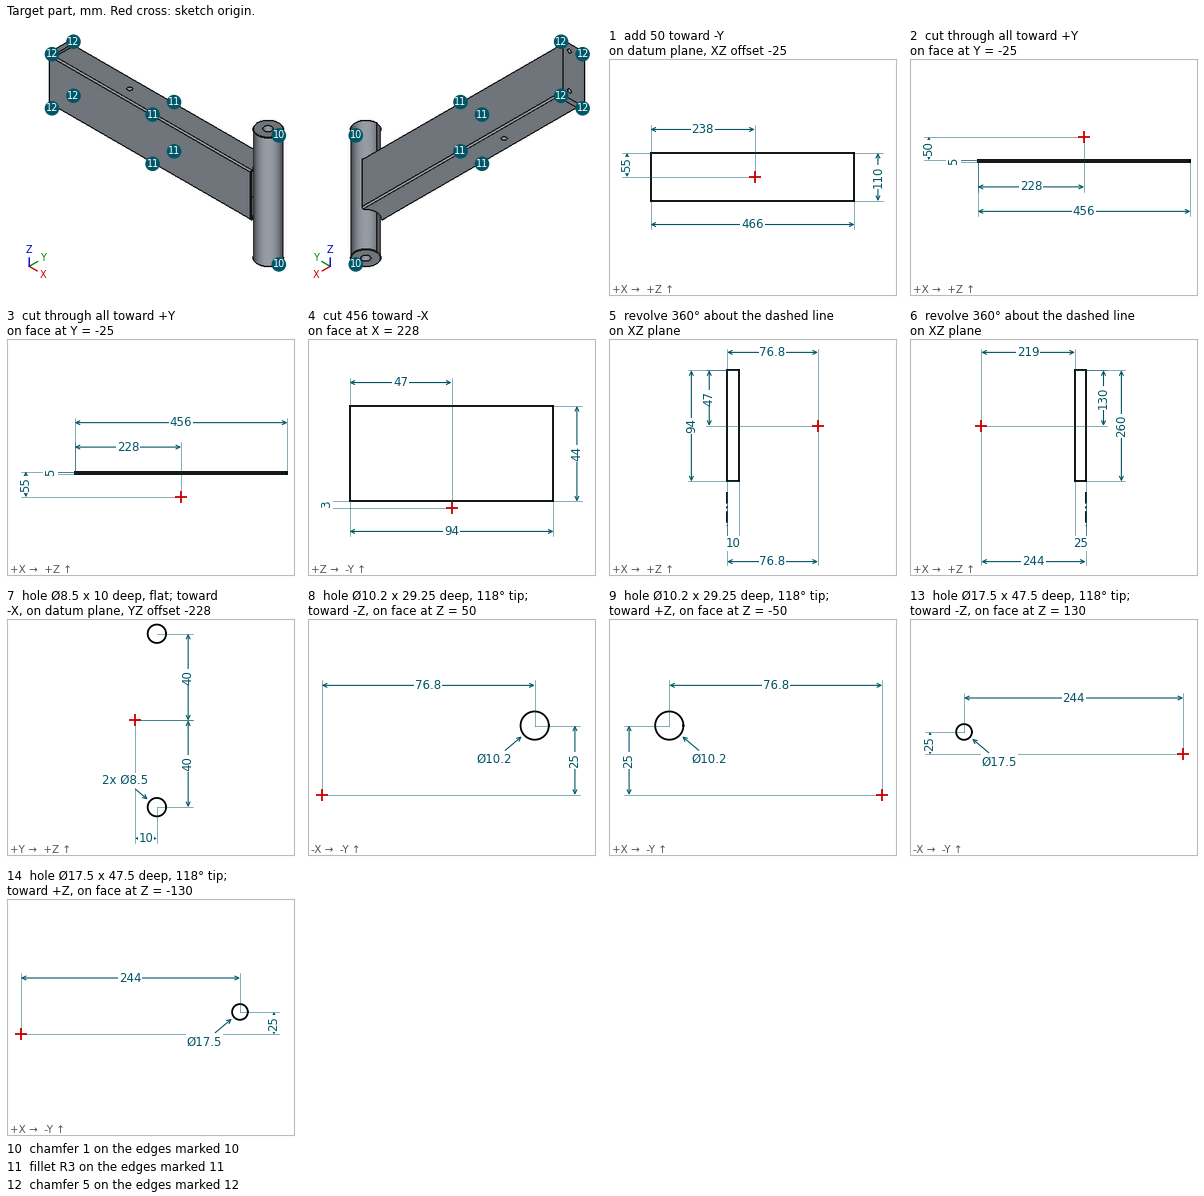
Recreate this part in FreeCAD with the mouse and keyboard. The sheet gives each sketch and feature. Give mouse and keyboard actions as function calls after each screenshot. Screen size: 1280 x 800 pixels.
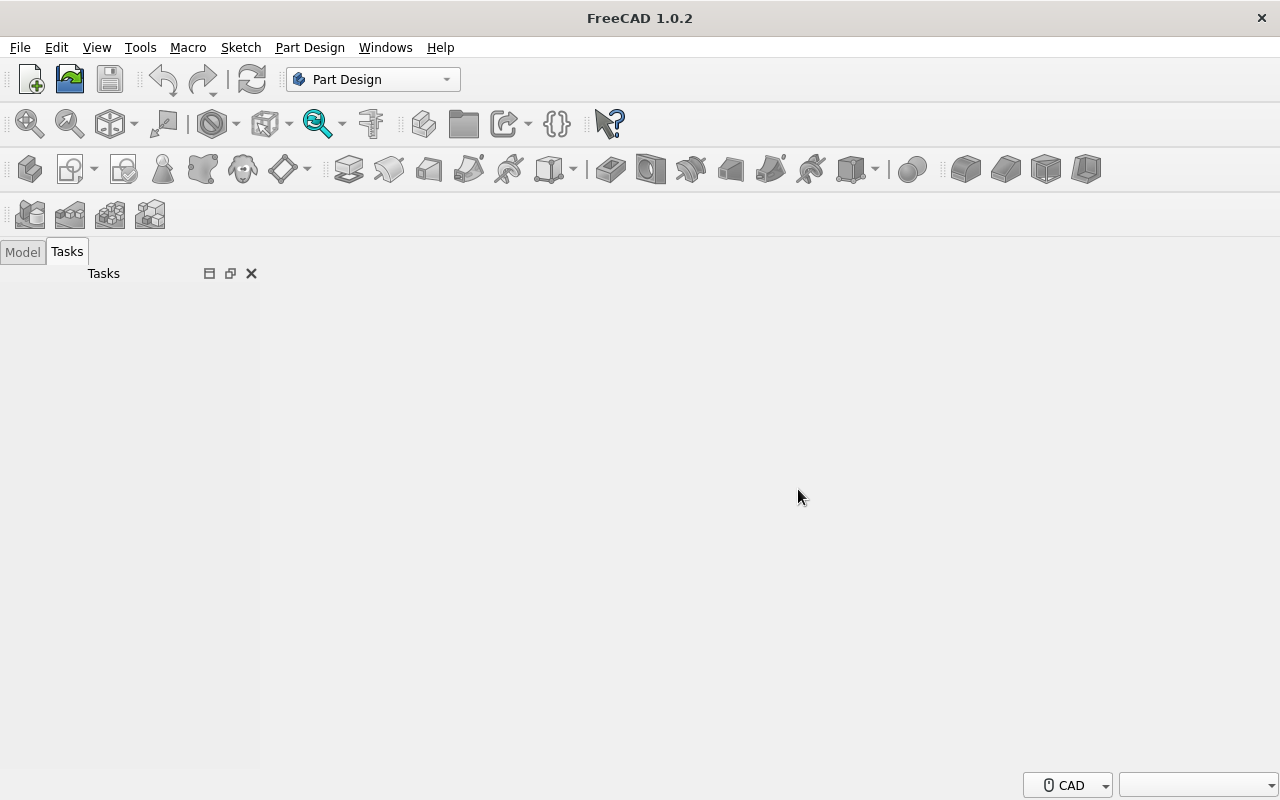
click(30, 80)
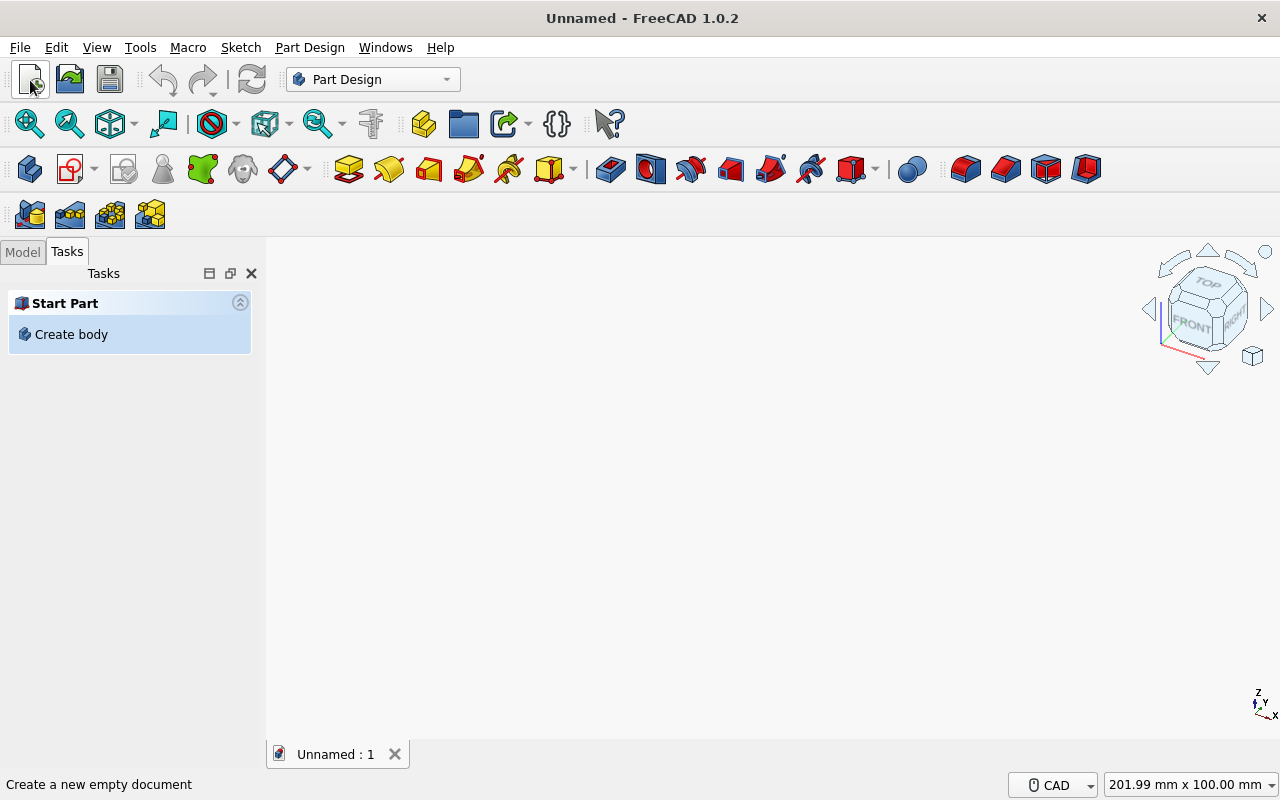
click(30, 170)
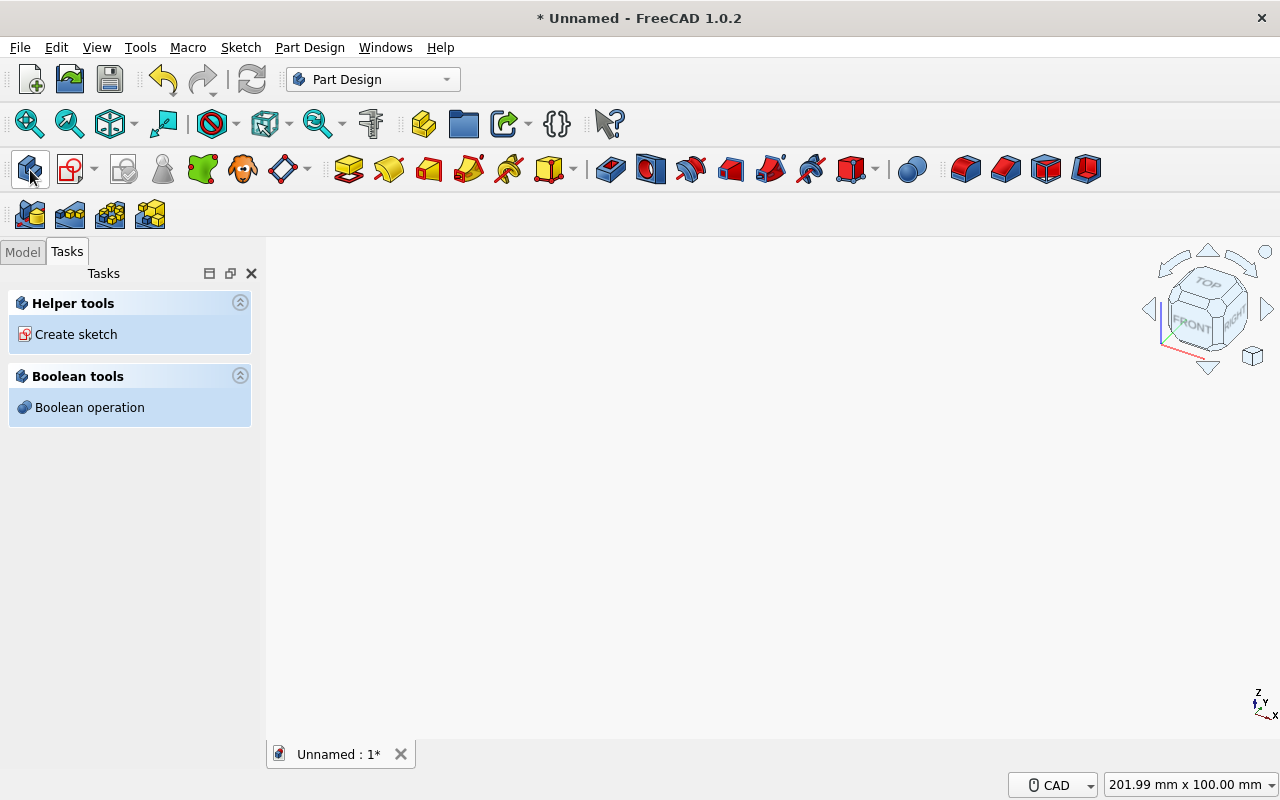
click(23, 251)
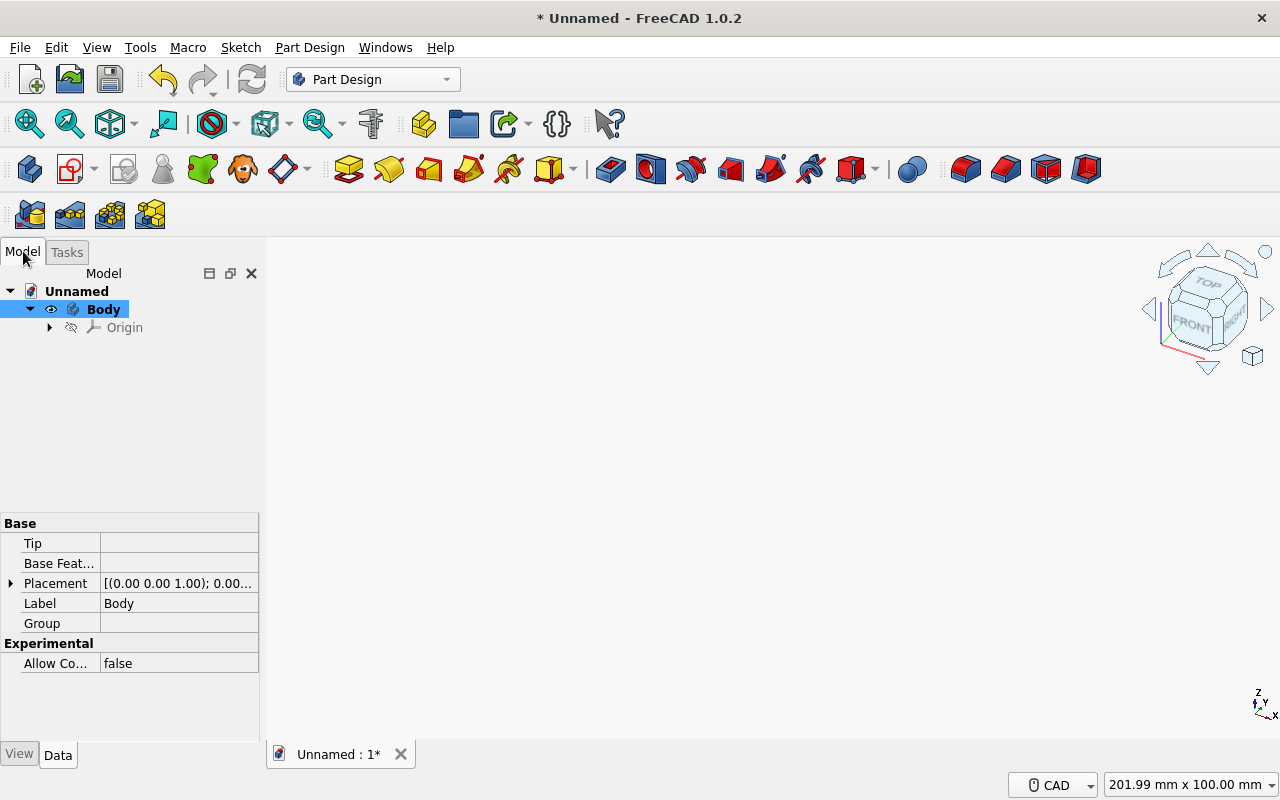
click(50, 327)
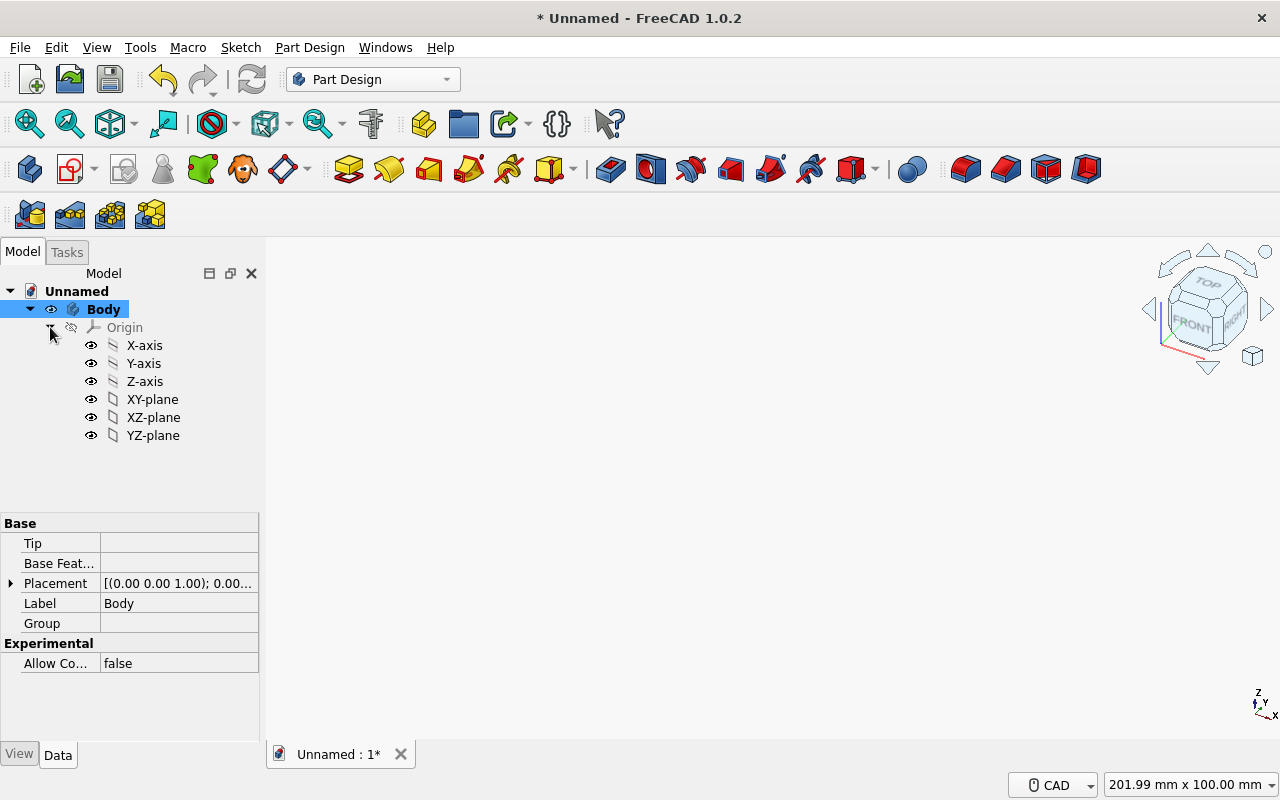
click(136, 417)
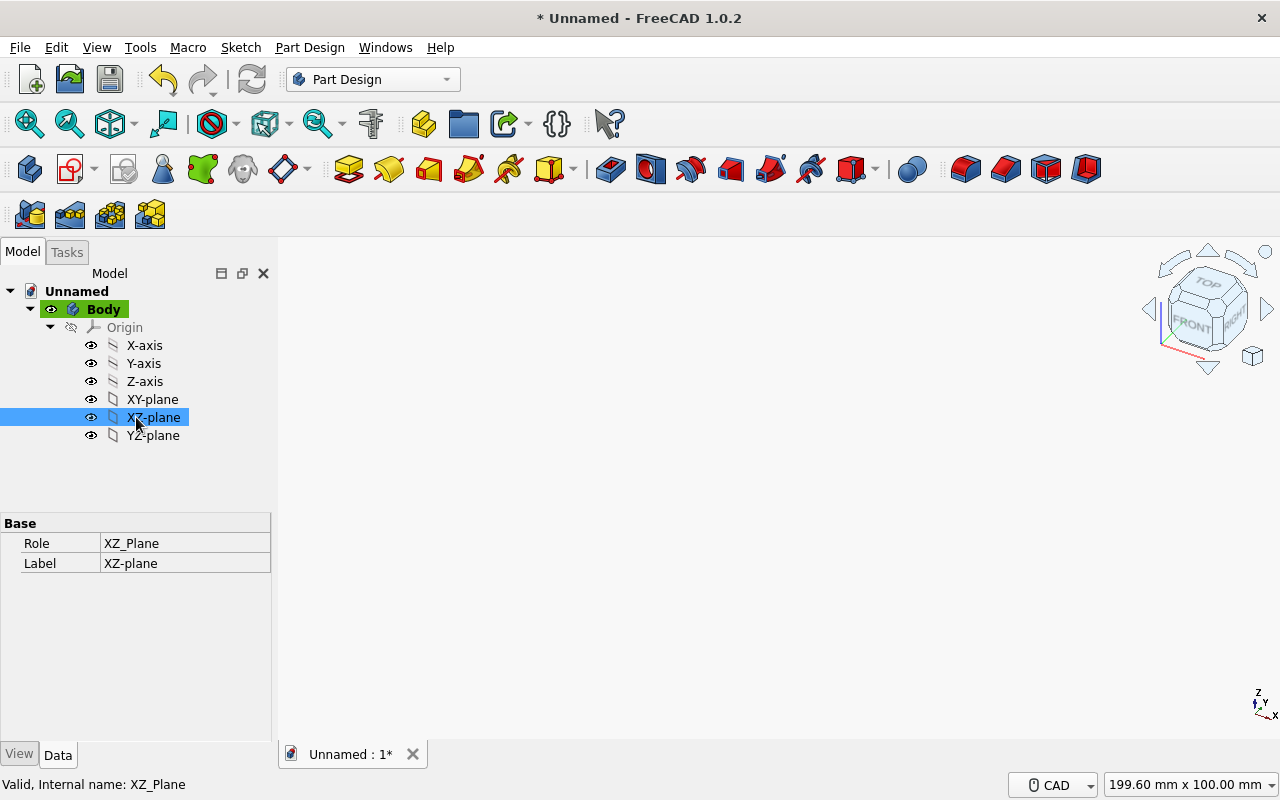
click(284, 170)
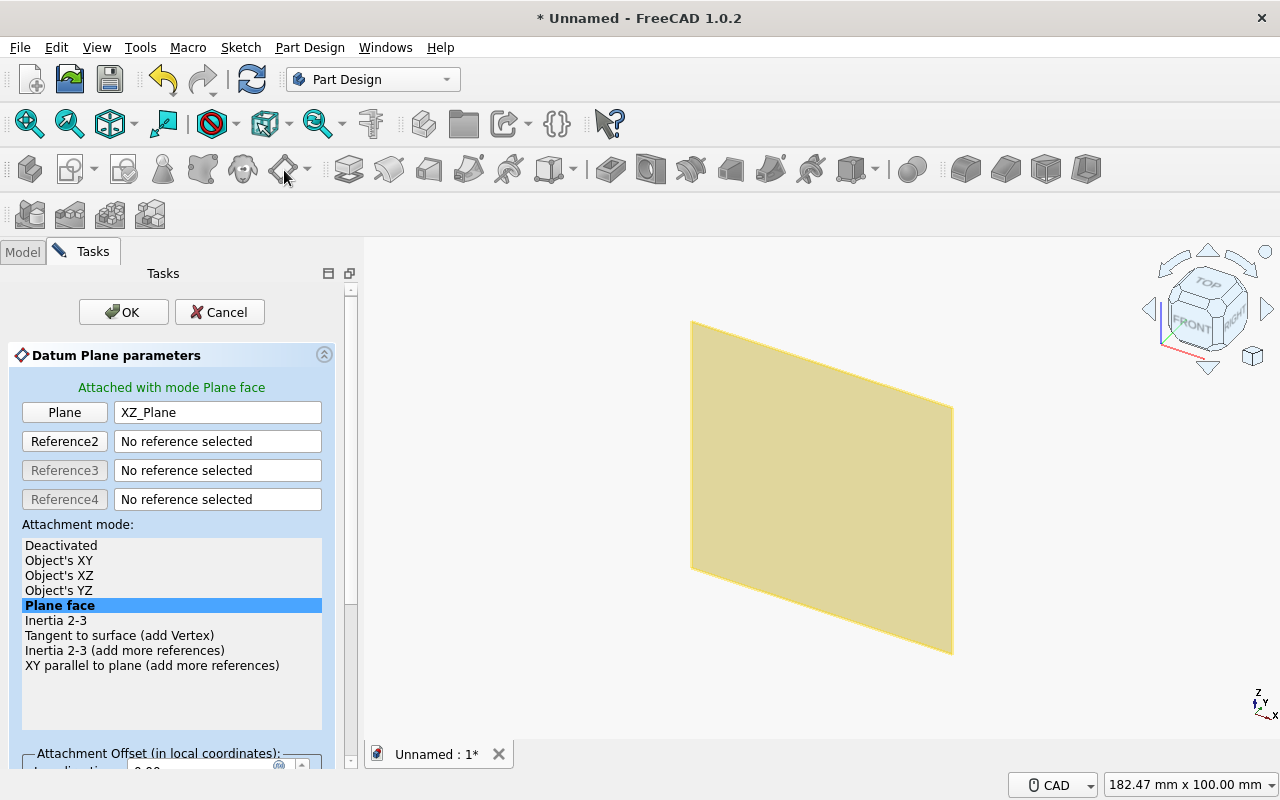
scroll(351, 526, down, 3)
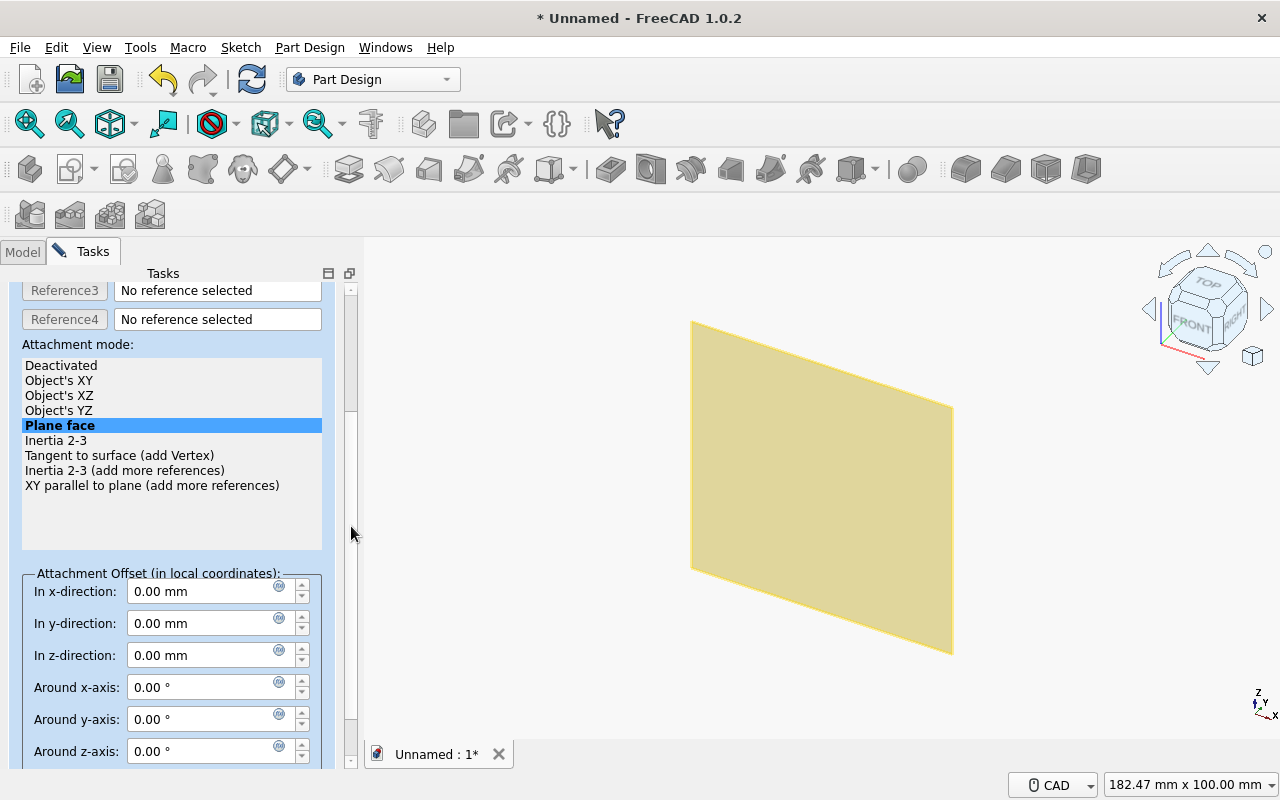
triple_click(210, 655)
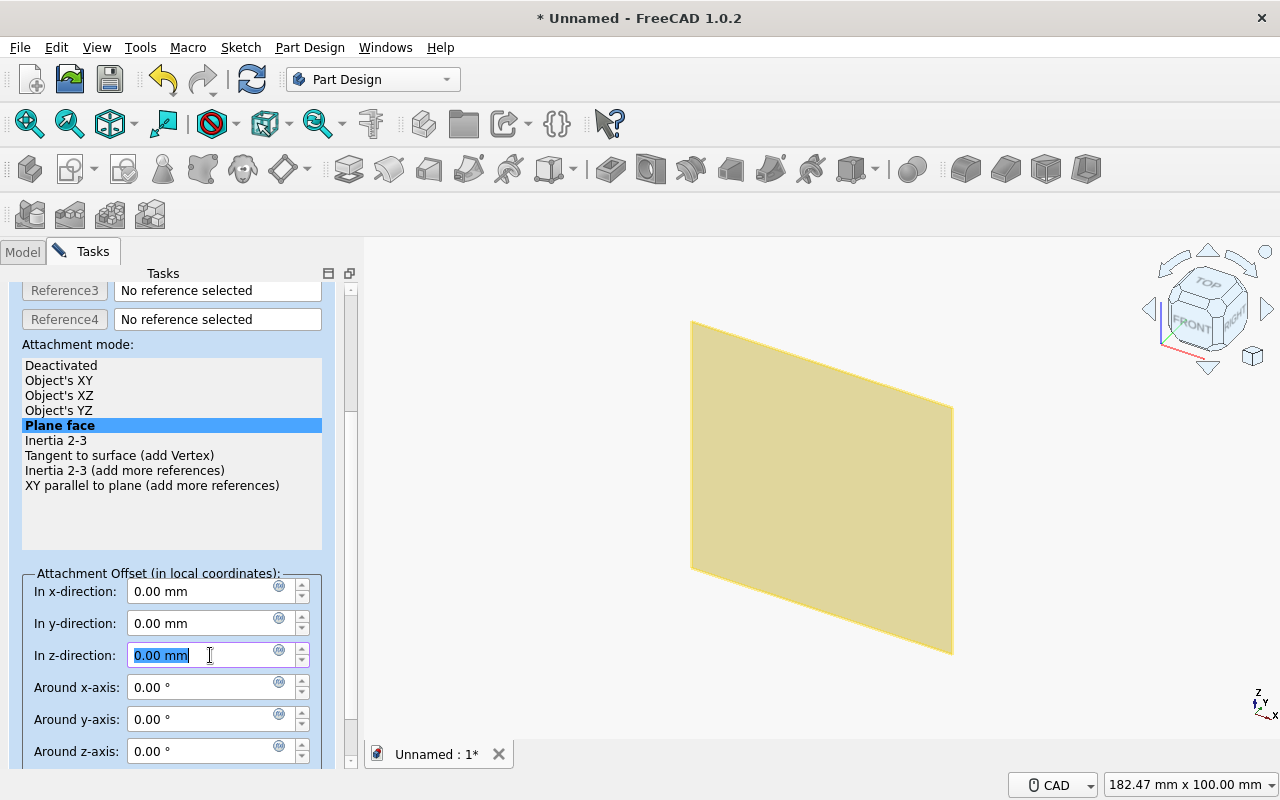
text(-25)
key(Tab)